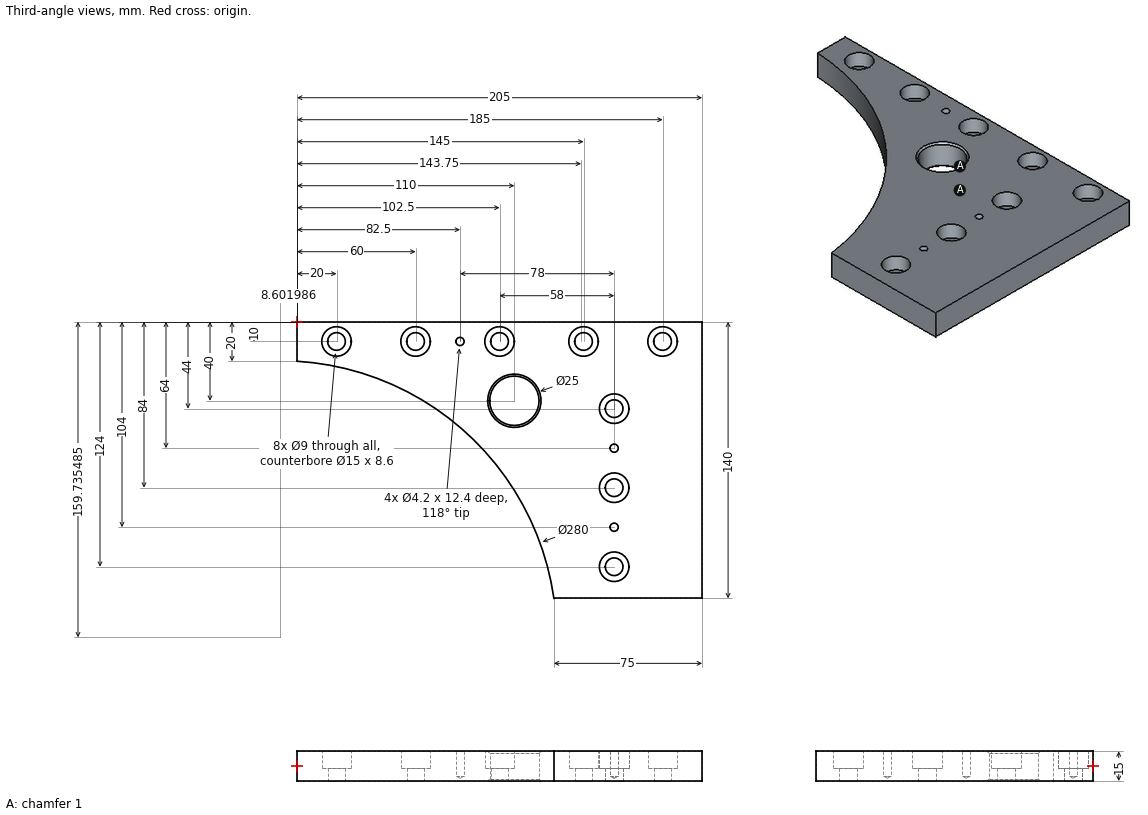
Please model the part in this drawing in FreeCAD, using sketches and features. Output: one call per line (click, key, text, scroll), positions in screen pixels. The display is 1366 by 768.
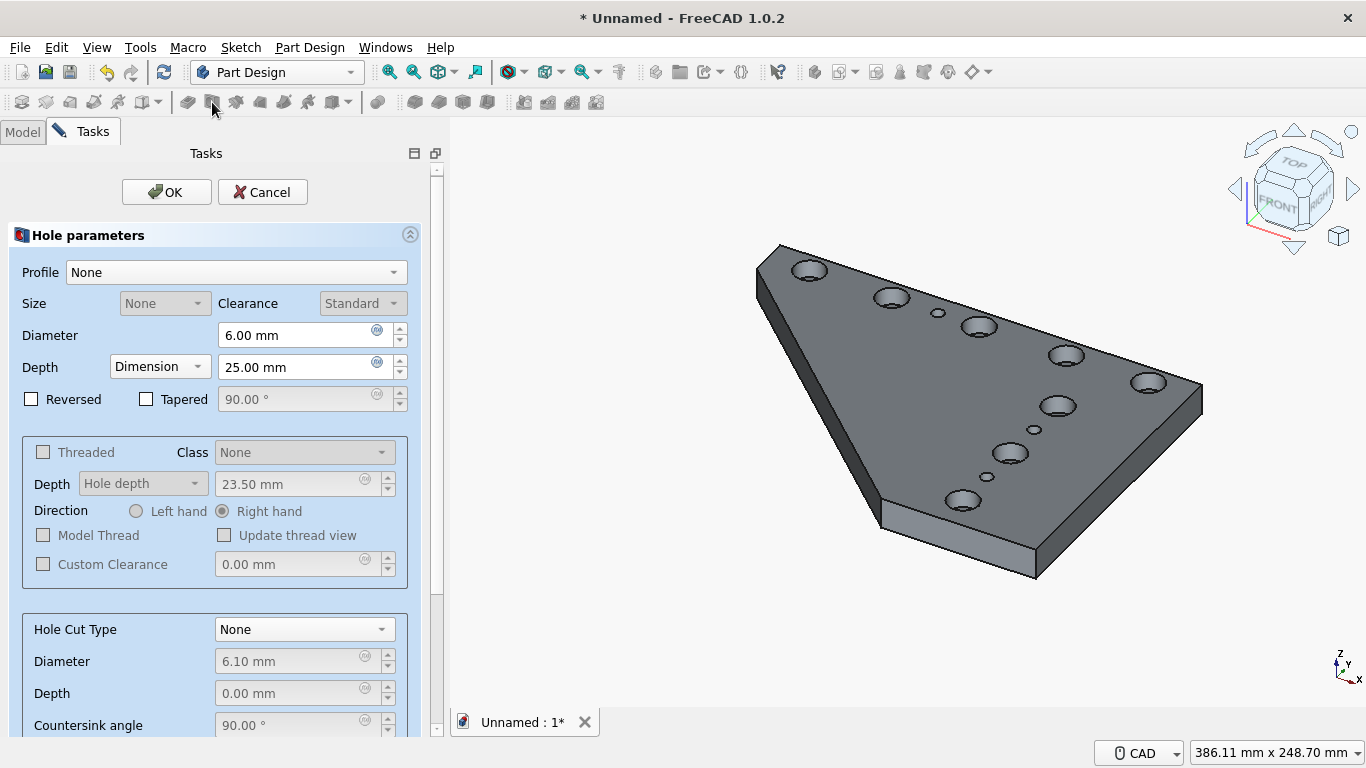
triple_click(305, 335)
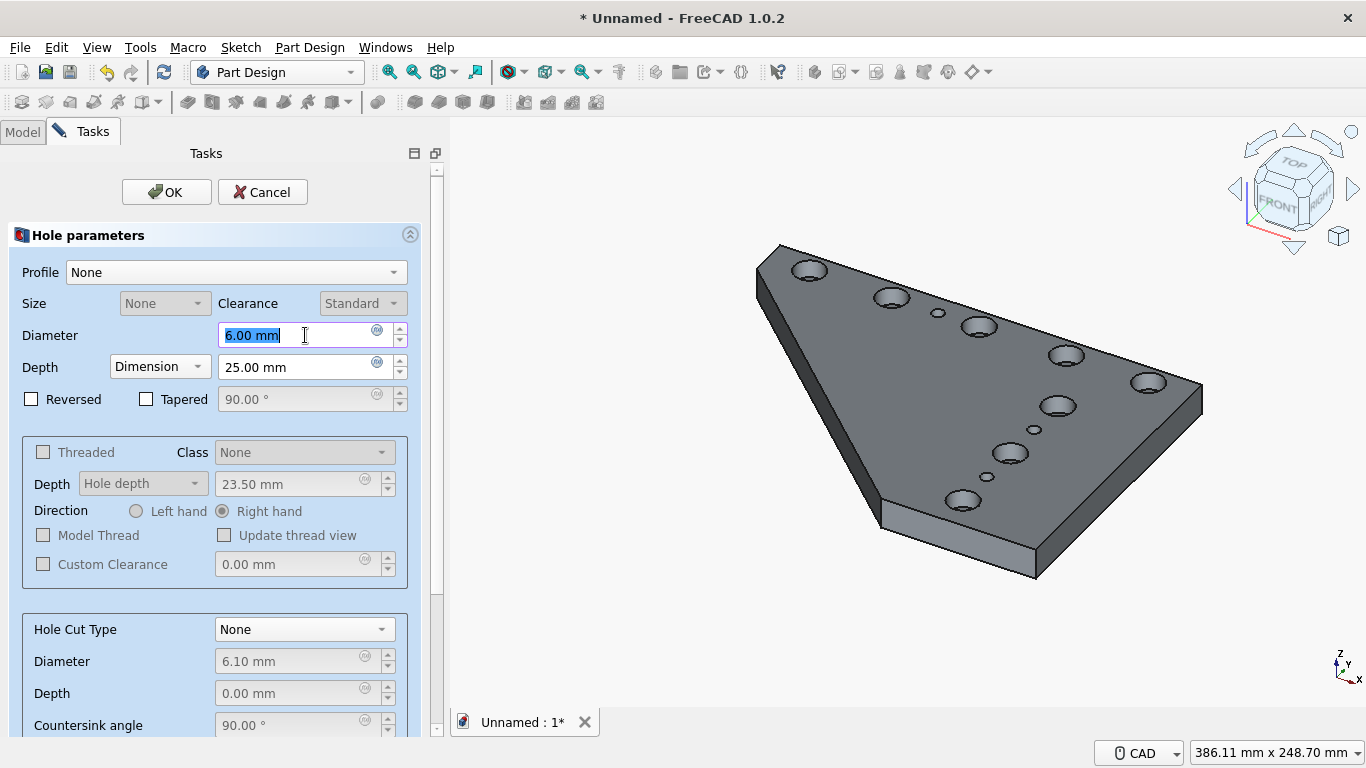
text(4.2)
key(Tab)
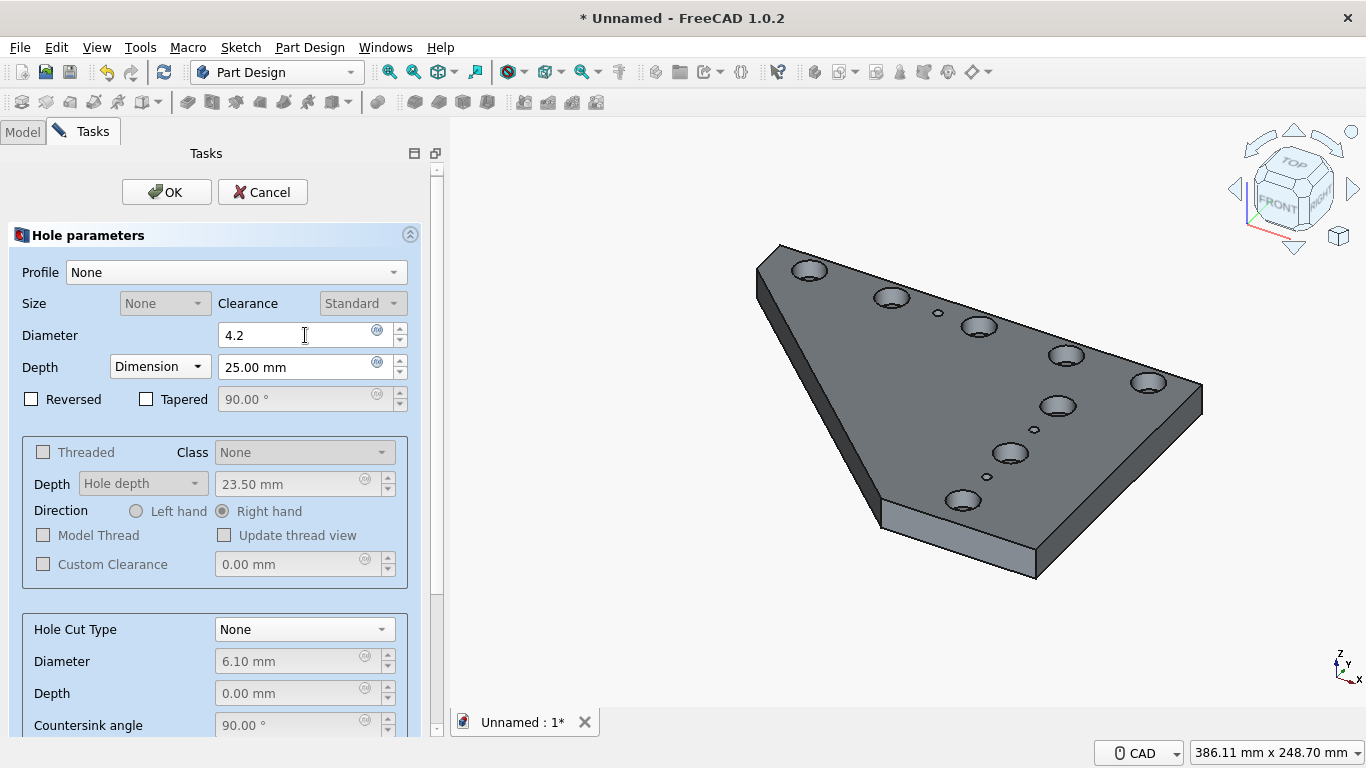
triple_click(305, 367)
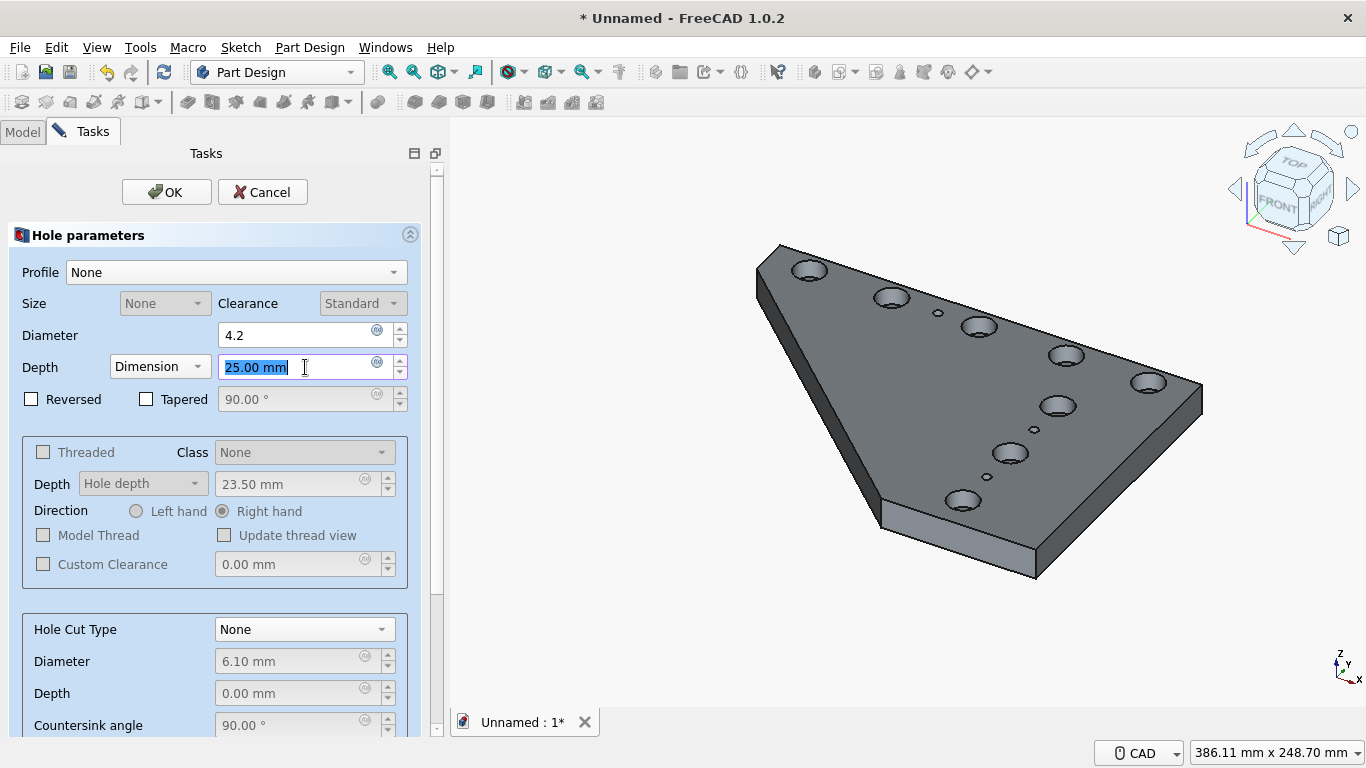
text(12.4)
key(Tab)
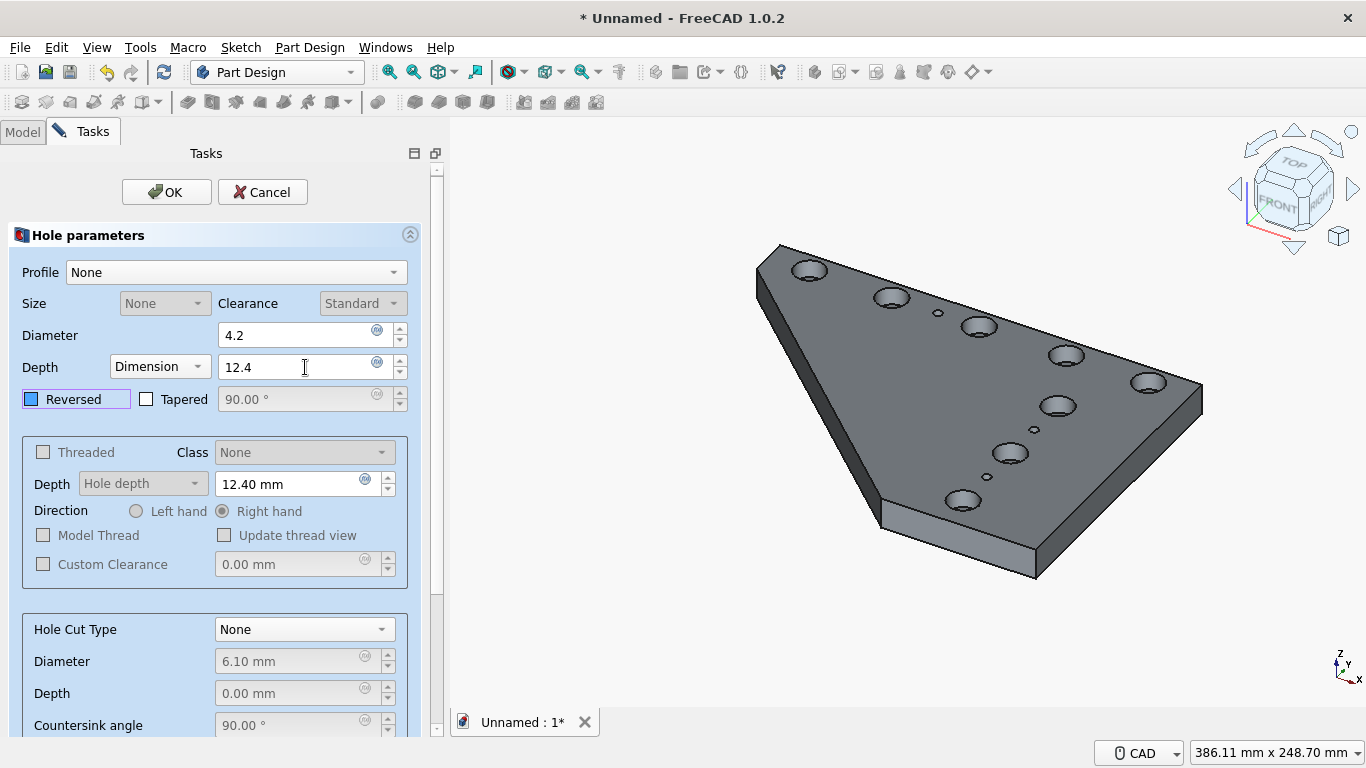
click(167, 192)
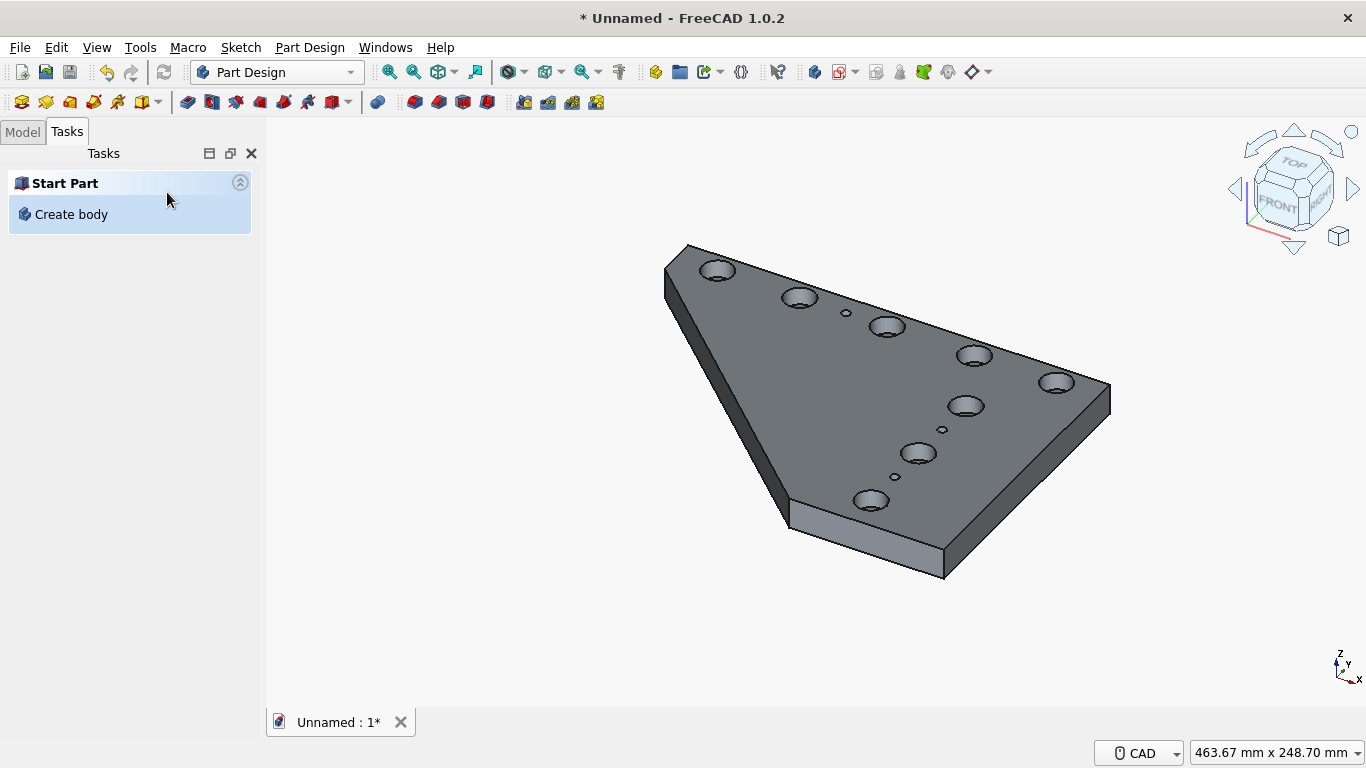
click(816, 396)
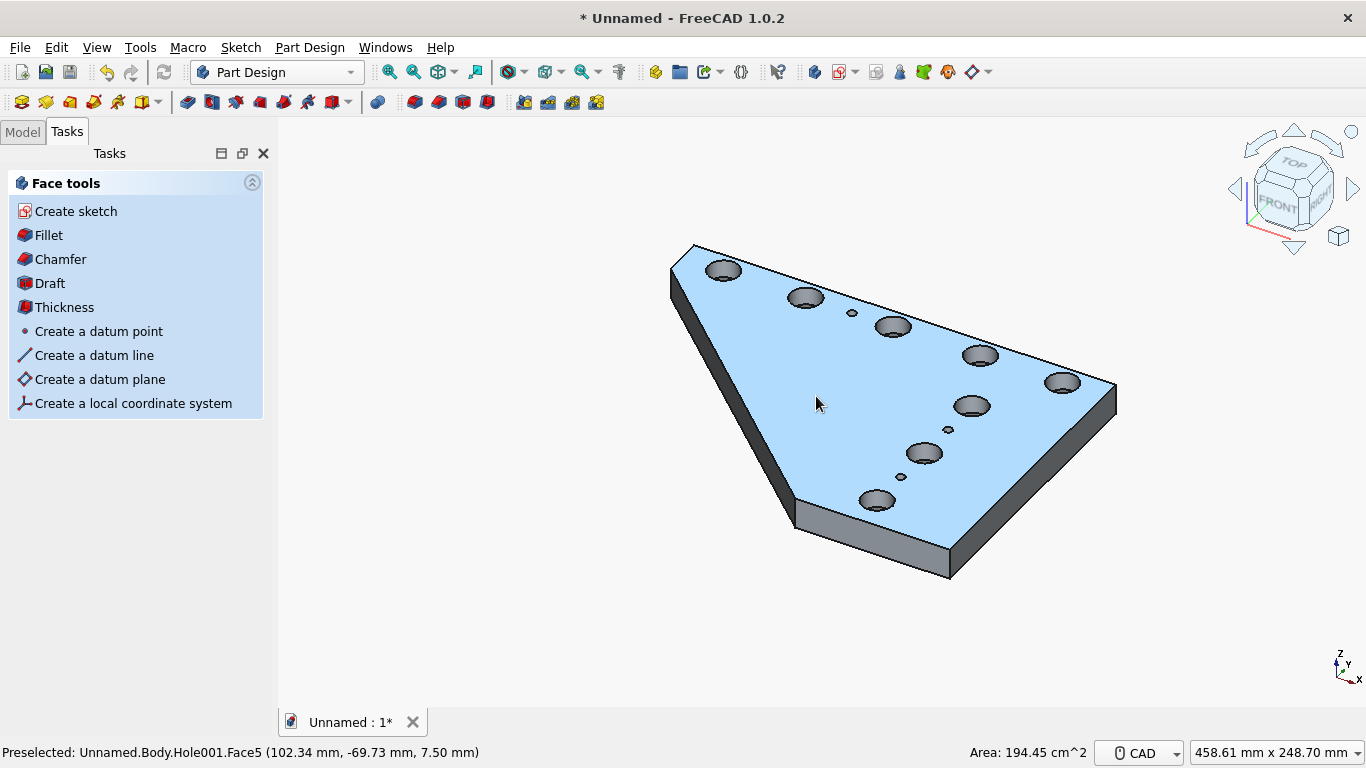
click(840, 72)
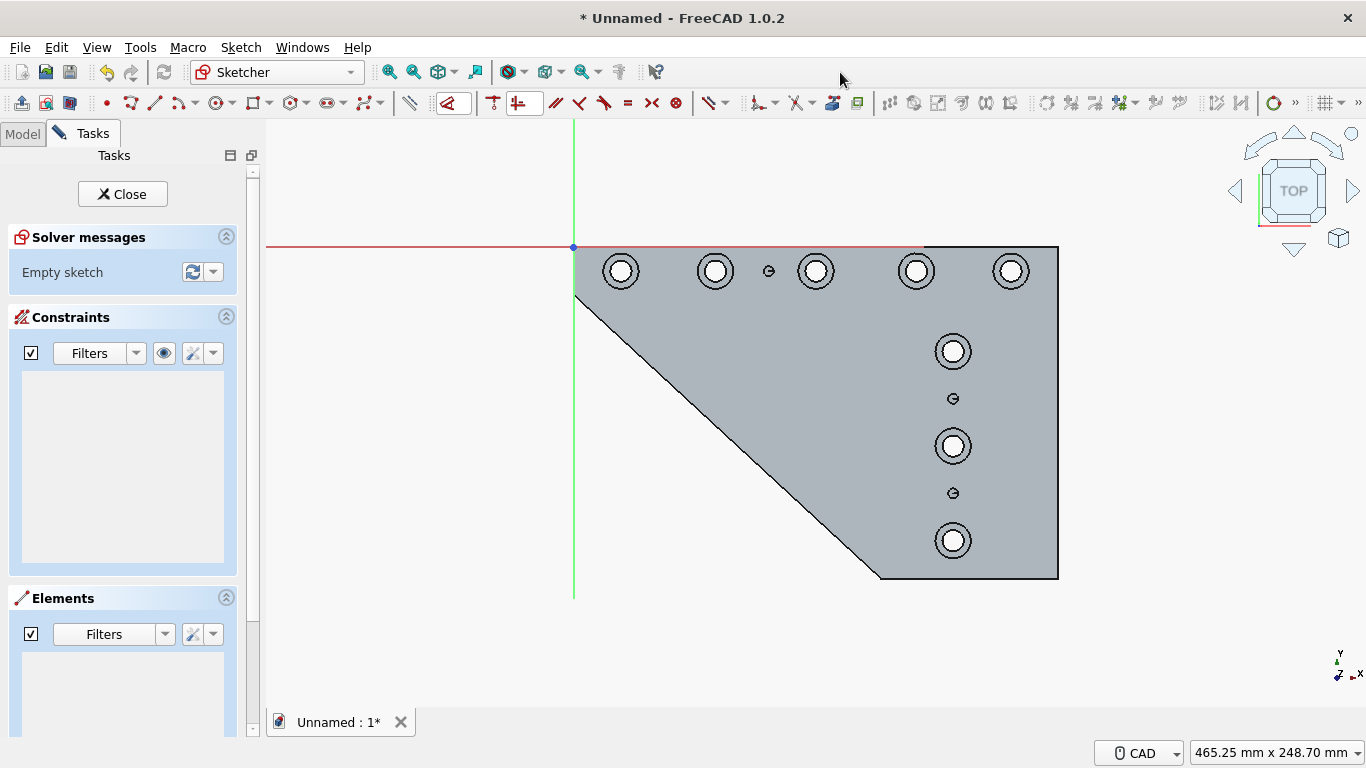
scroll(984, 183, down, 3)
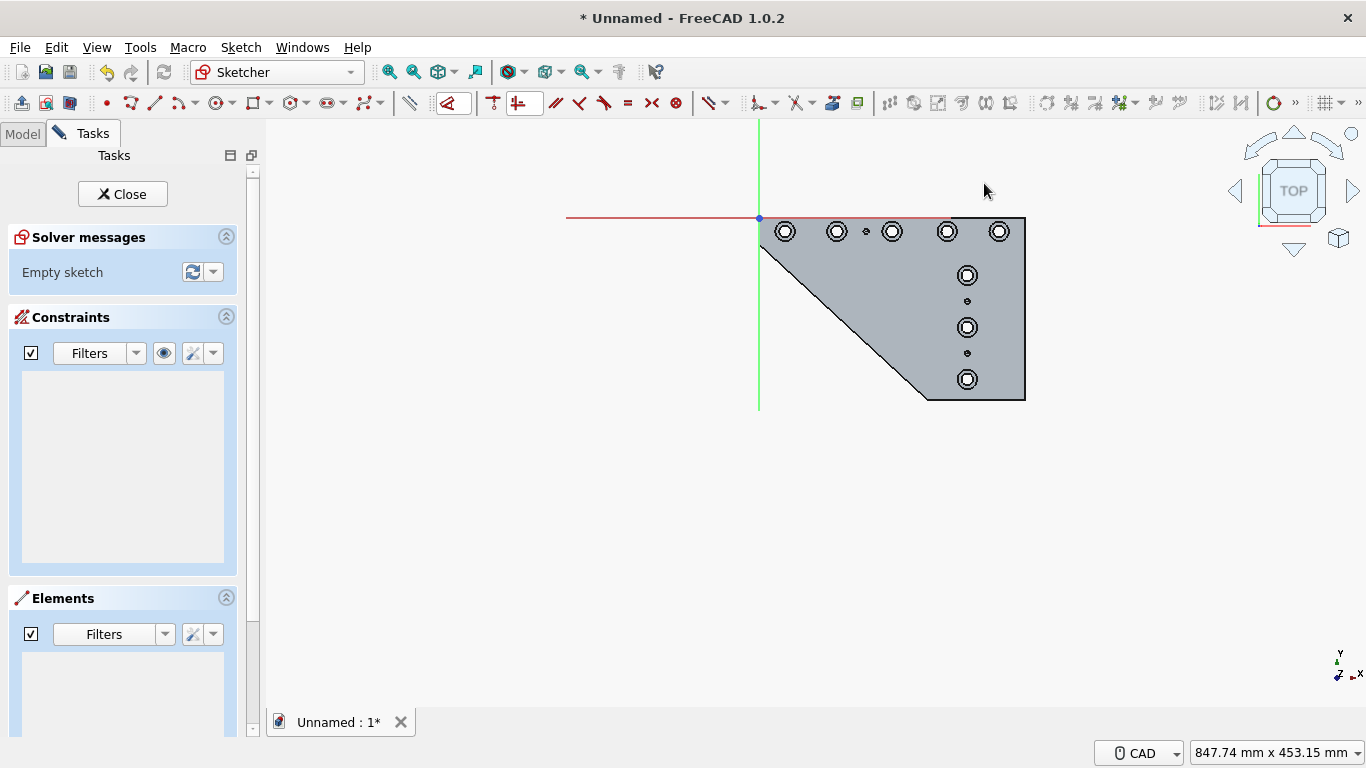
click(216, 104)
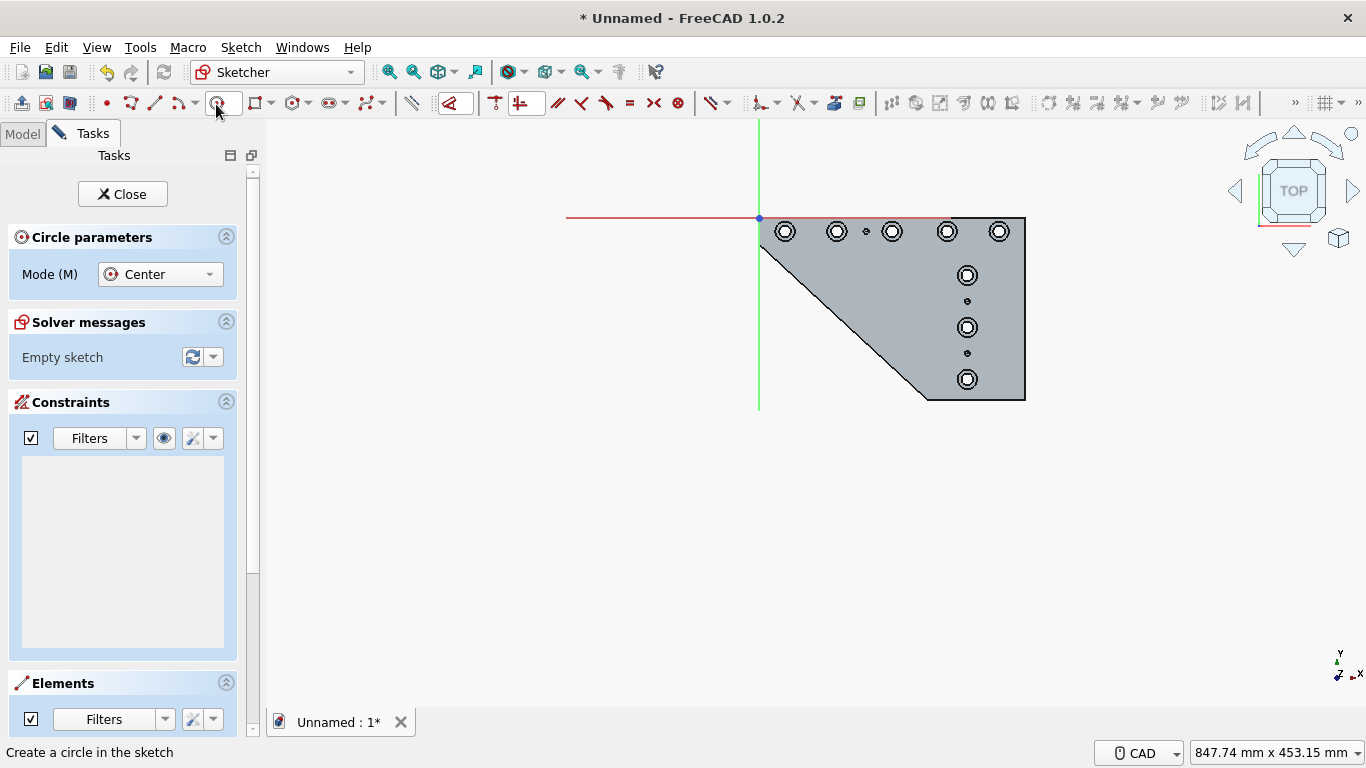
scroll(748, 426, up, 2)